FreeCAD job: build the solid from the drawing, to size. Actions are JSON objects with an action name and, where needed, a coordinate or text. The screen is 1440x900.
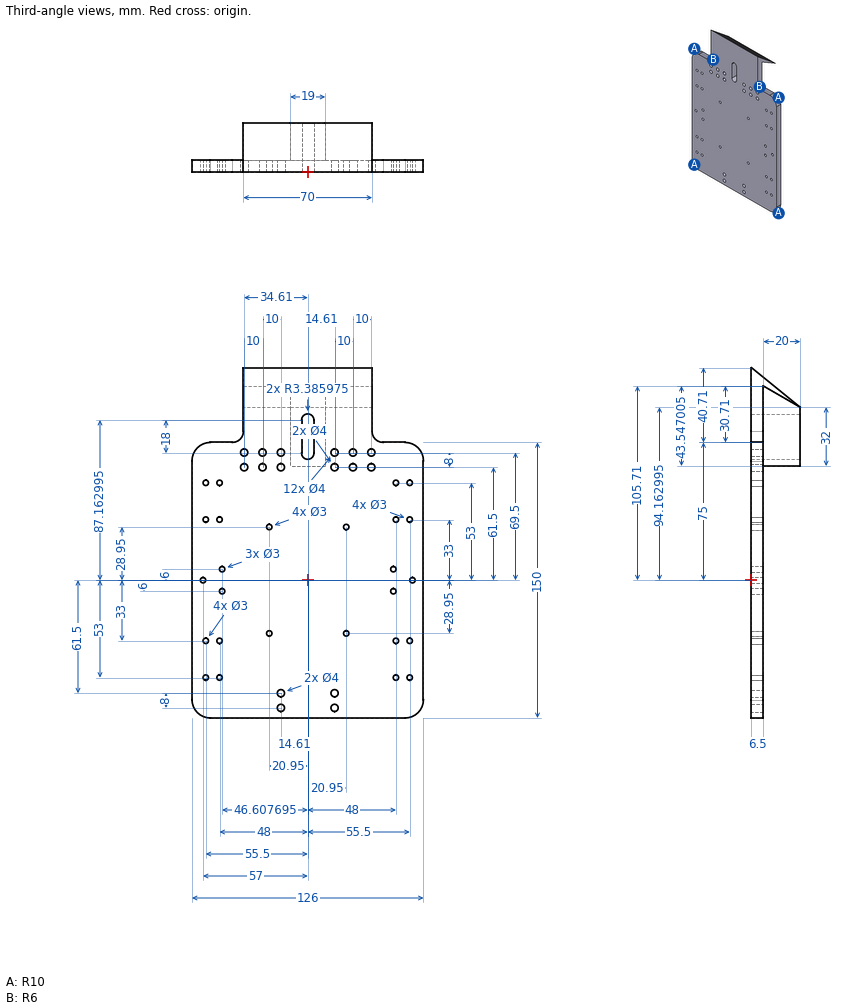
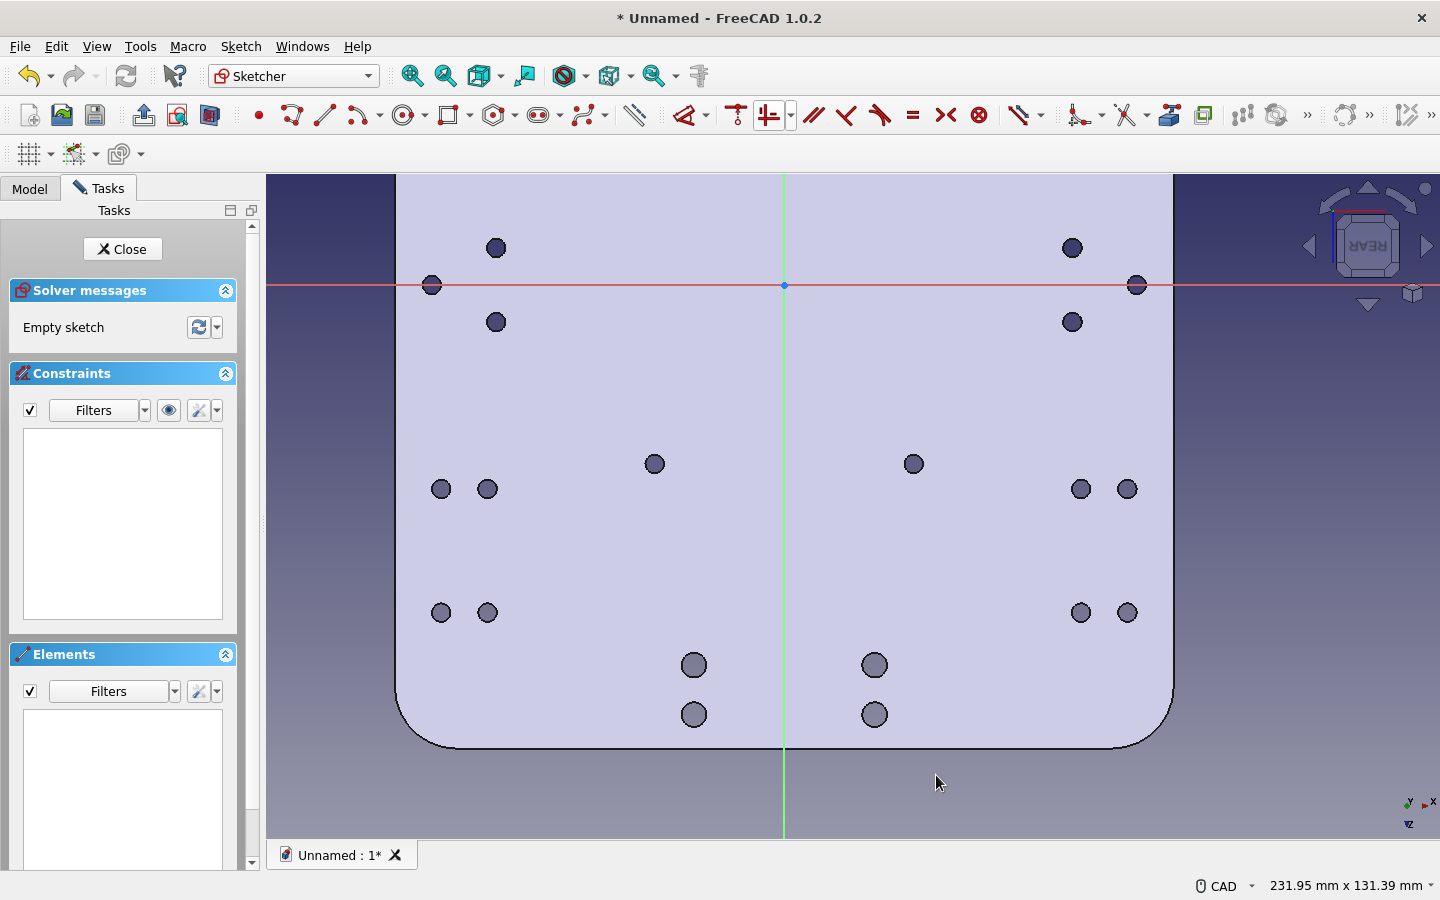
{"action": "left_click", "coordinate": [402, 116]}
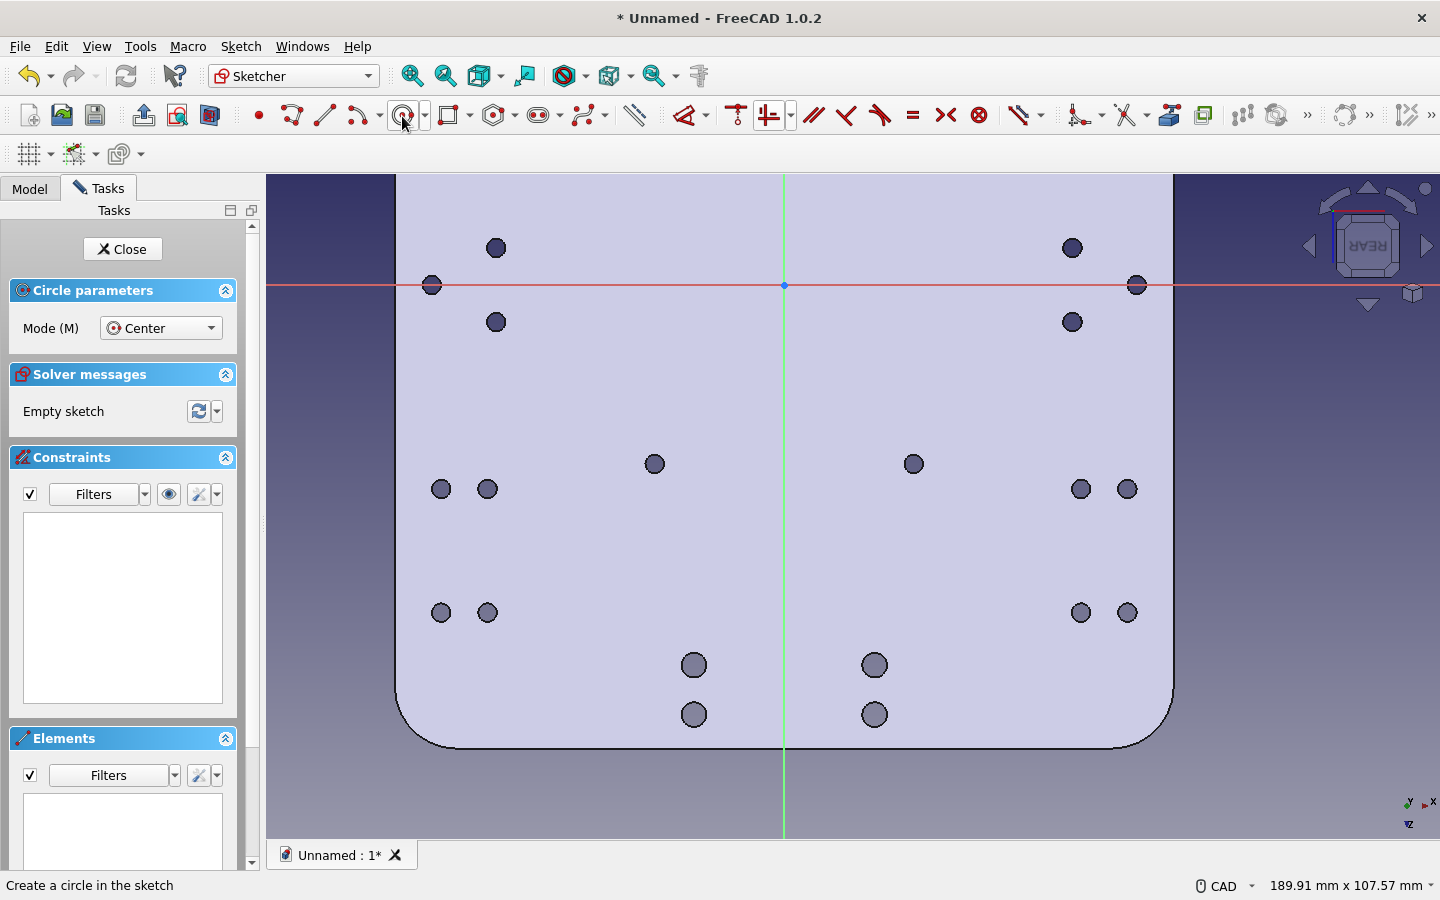
{"action": "scroll", "coordinate": [875, 715], "scroll_direction": "up", "scroll_amount": 4}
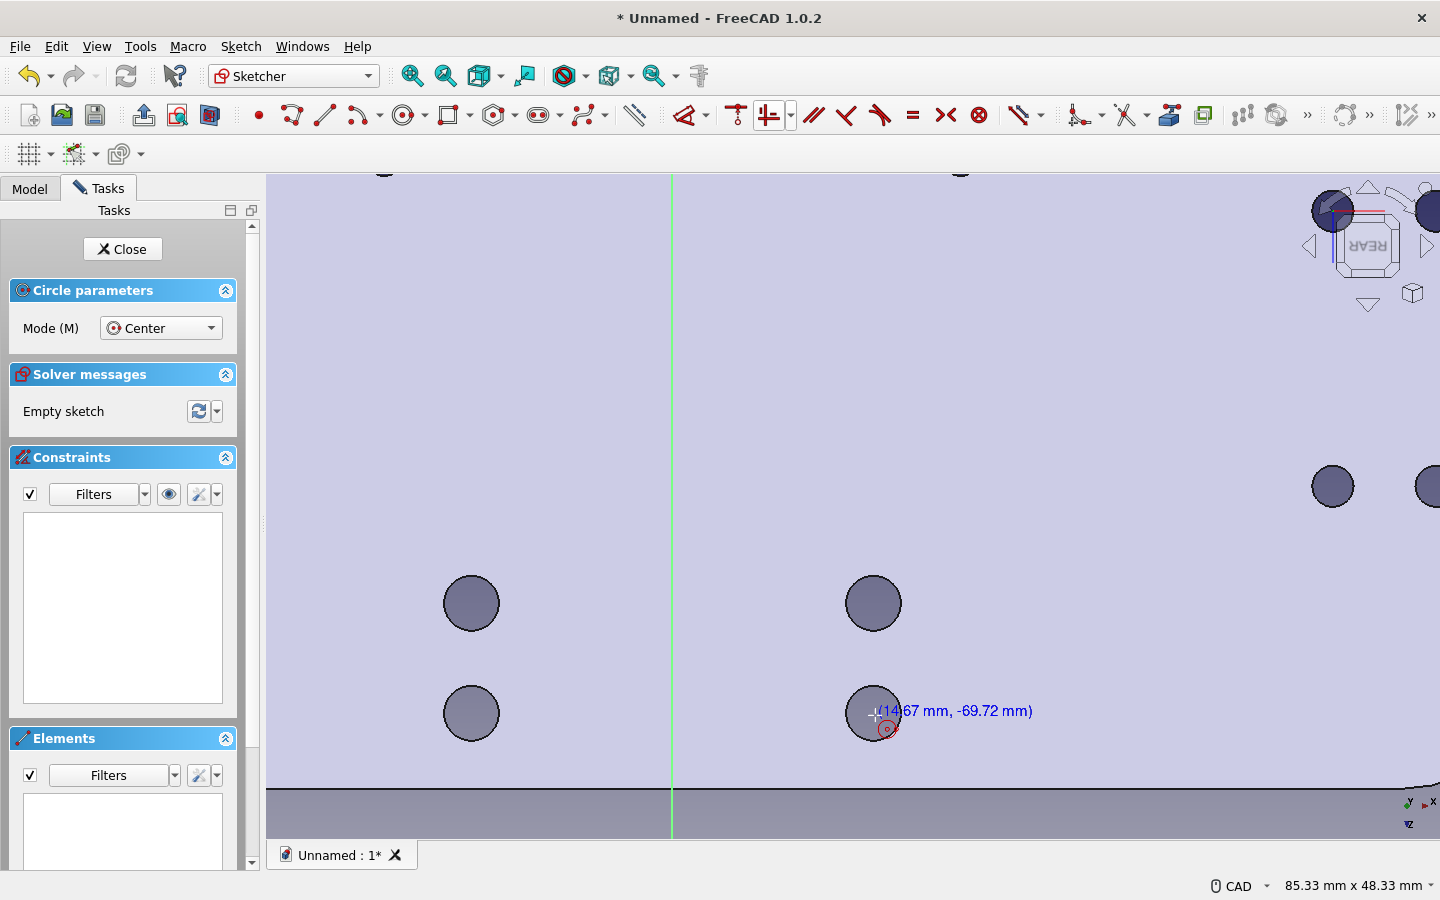
{"action": "left_click", "coordinate": [874, 713]}
{"action": "mouse_move", "coordinate": [893, 694]}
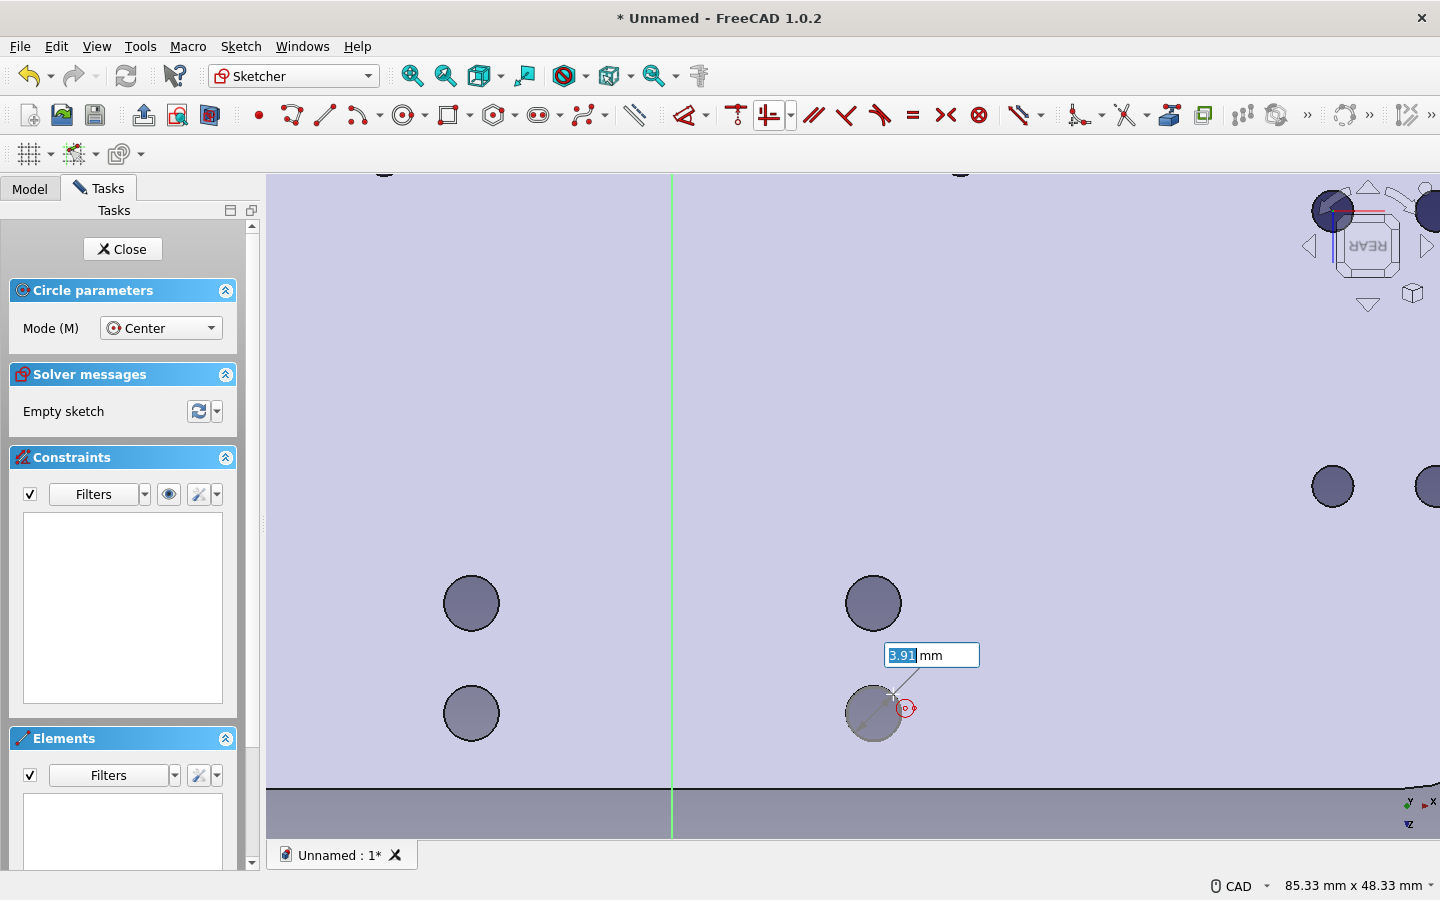
{"action": "type", "text": "4"}
{"action": "key", "text": "Return"}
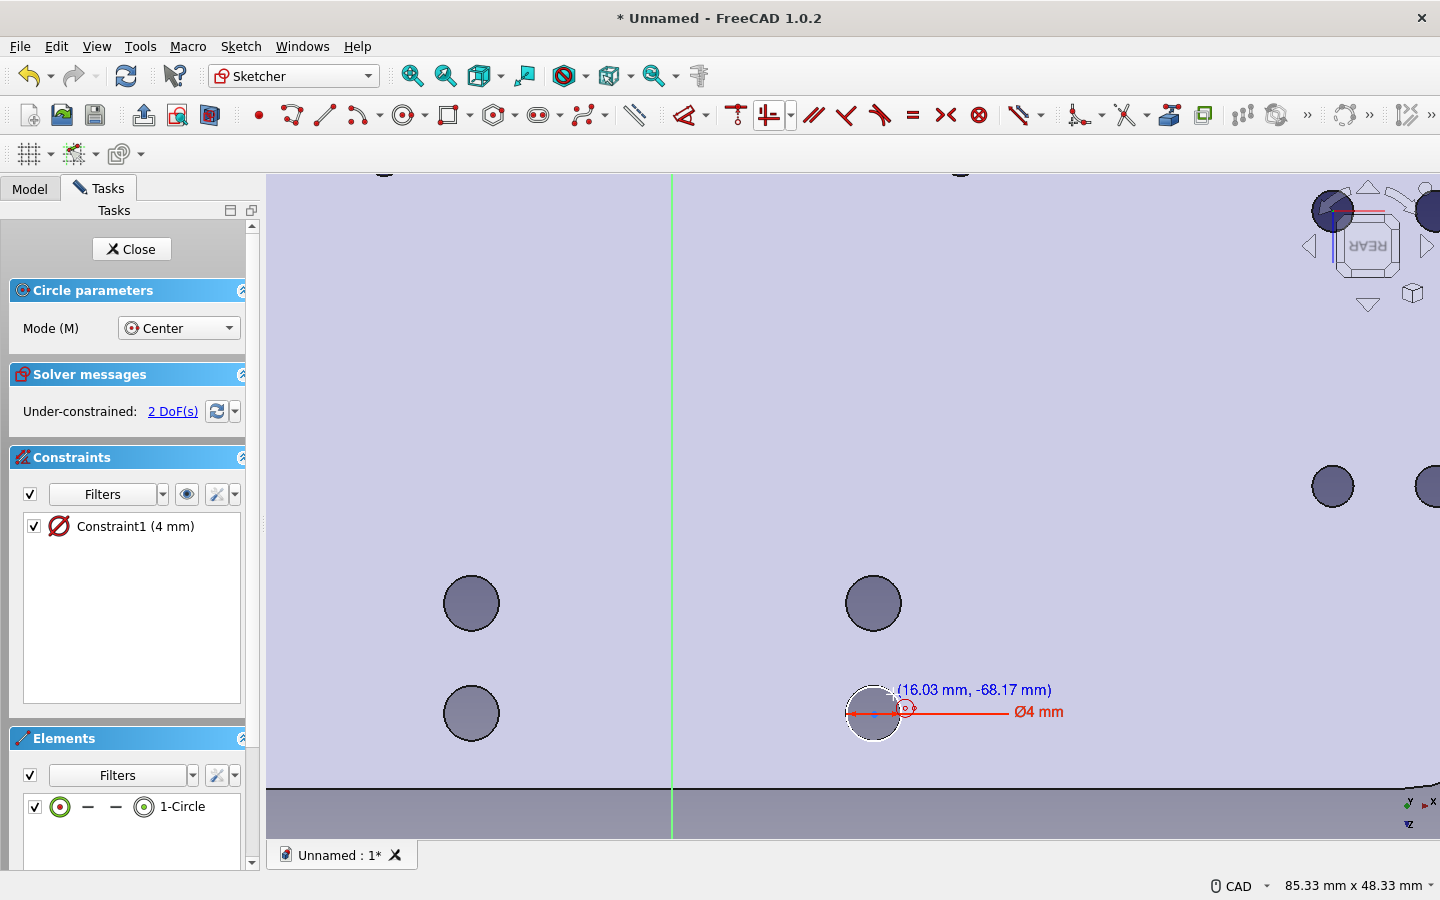
{"action": "left_click", "coordinate": [874, 603]}
{"action": "mouse_move", "coordinate": [893, 584]}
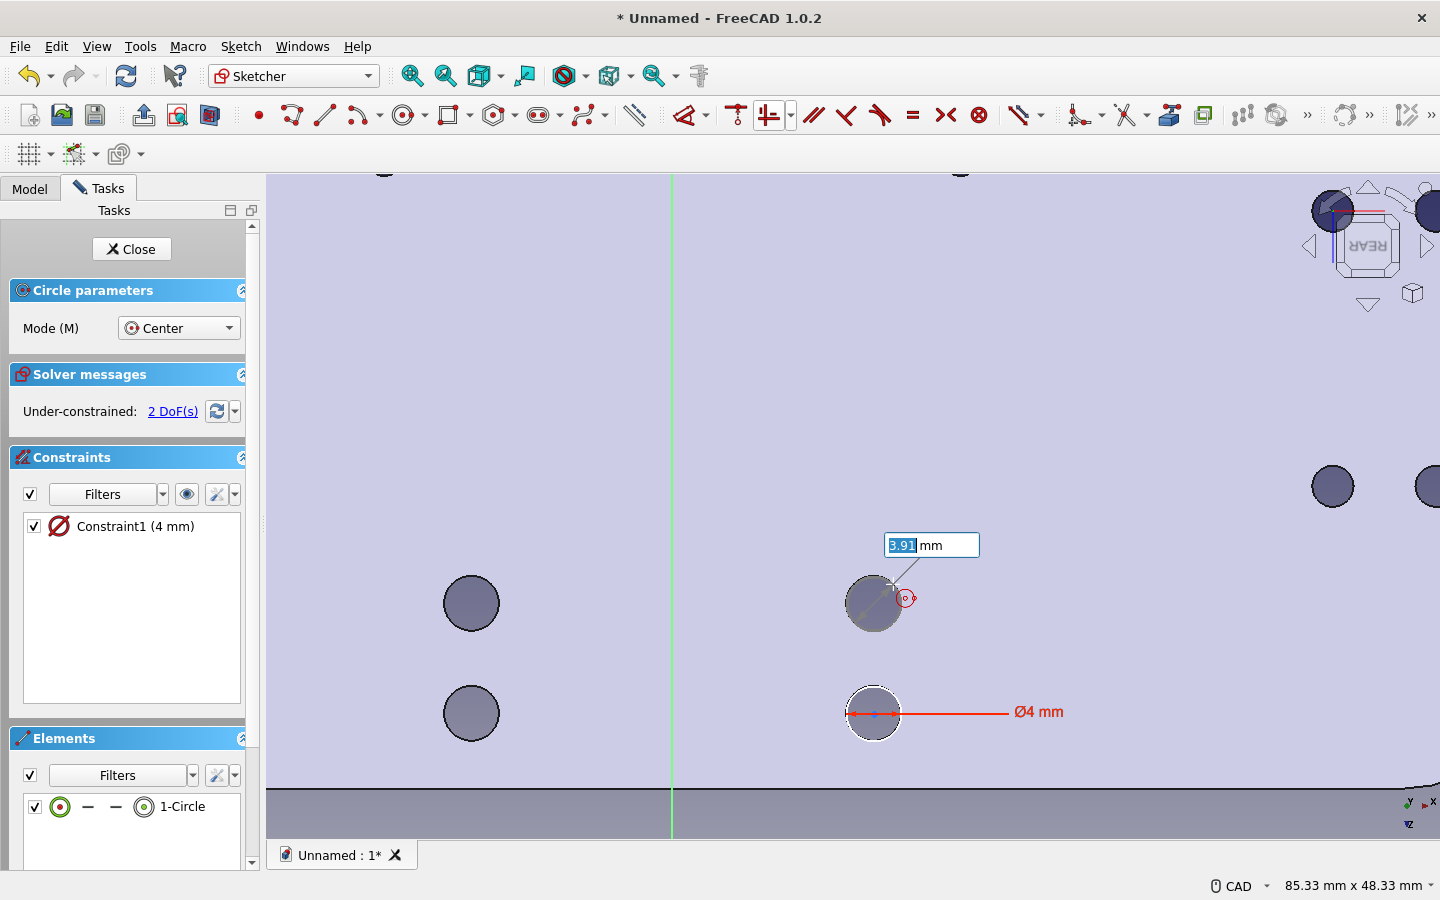
{"action": "type", "text": "4"}
{"action": "key", "text": "Return"}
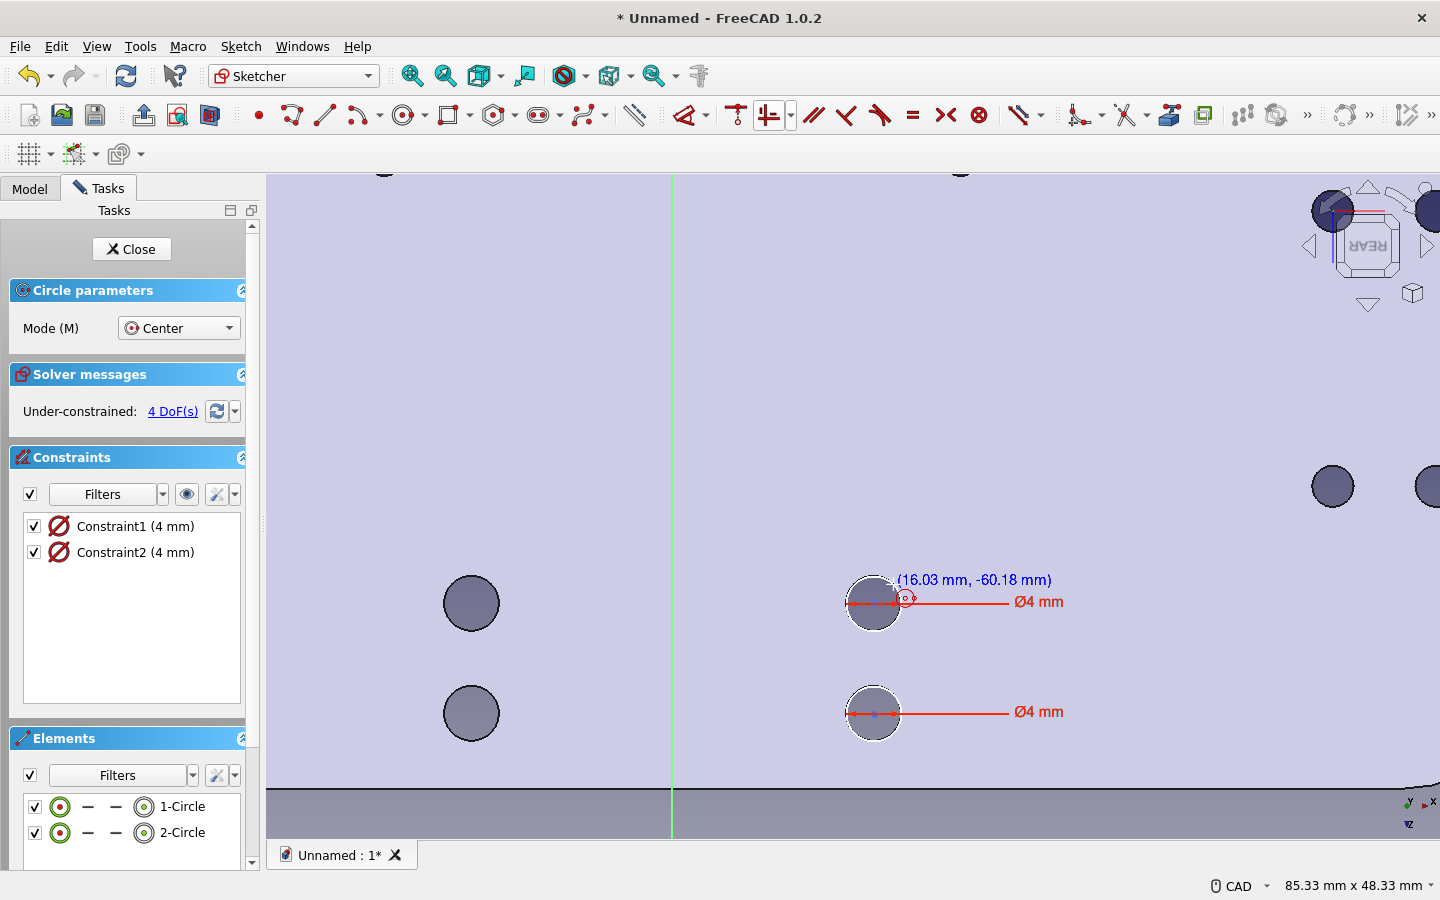
{"action": "left_click", "coordinate": [1011, 713]}
{"action": "mouse_move", "coordinate": [1031, 694]}